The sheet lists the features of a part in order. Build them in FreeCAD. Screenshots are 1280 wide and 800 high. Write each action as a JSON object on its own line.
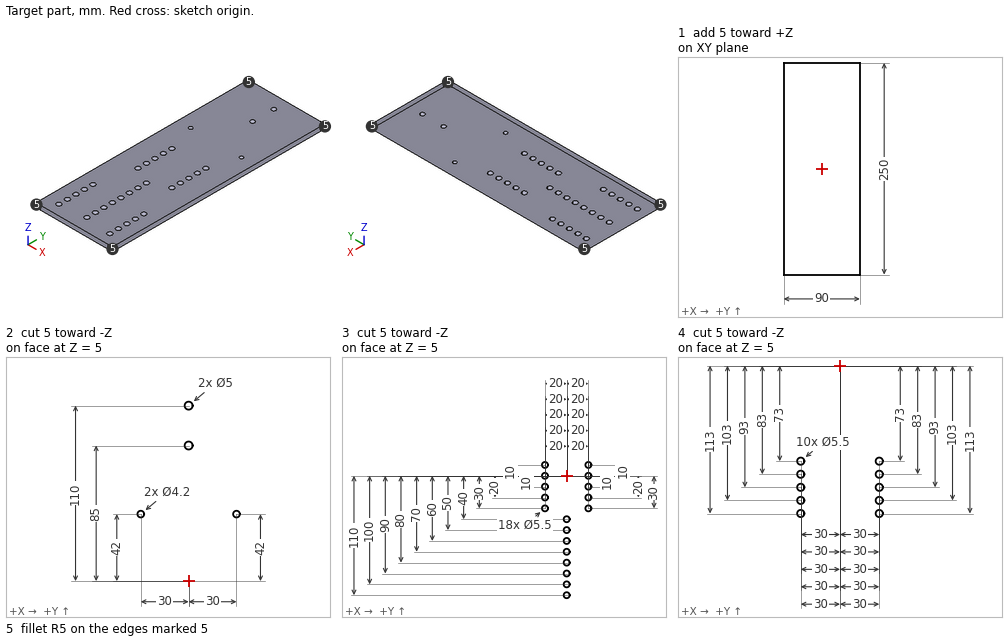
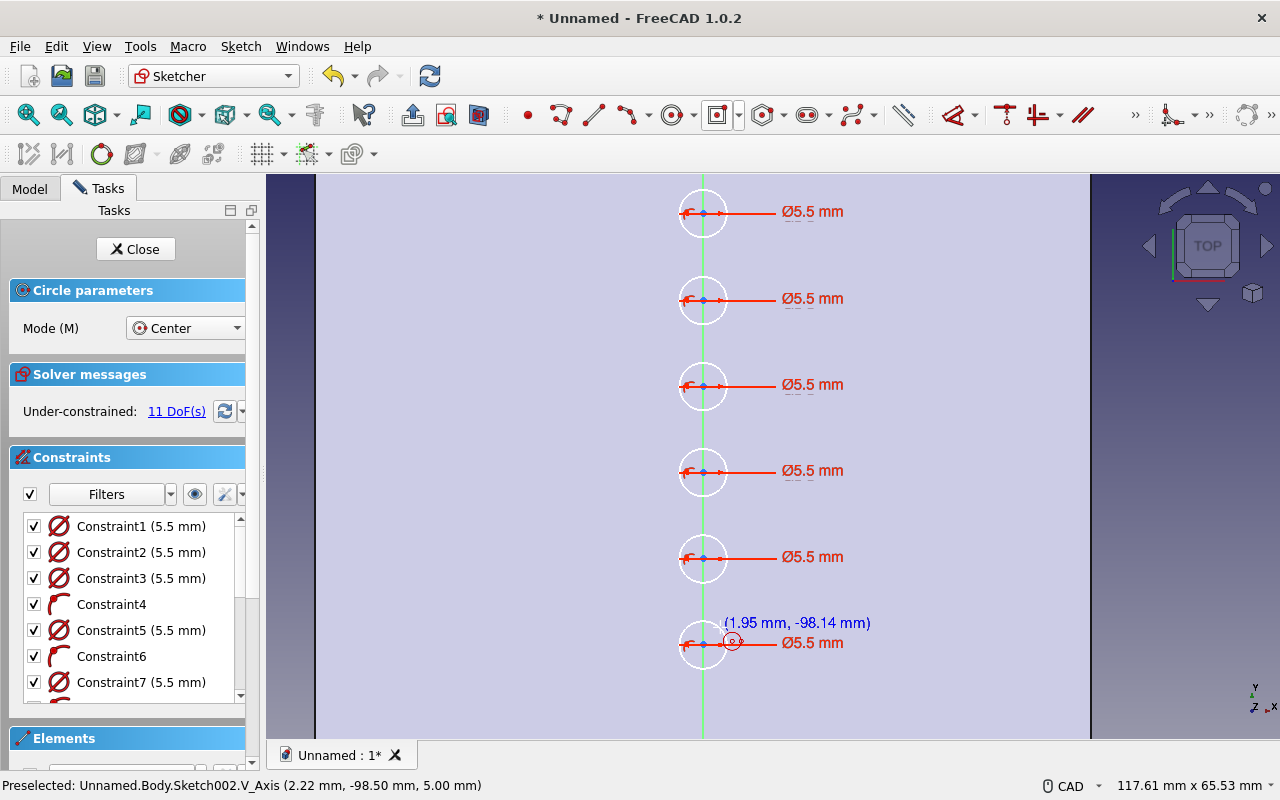
{"action": "scroll", "coordinate": [705, 561], "scroll_direction": "down", "scroll_amount": 6}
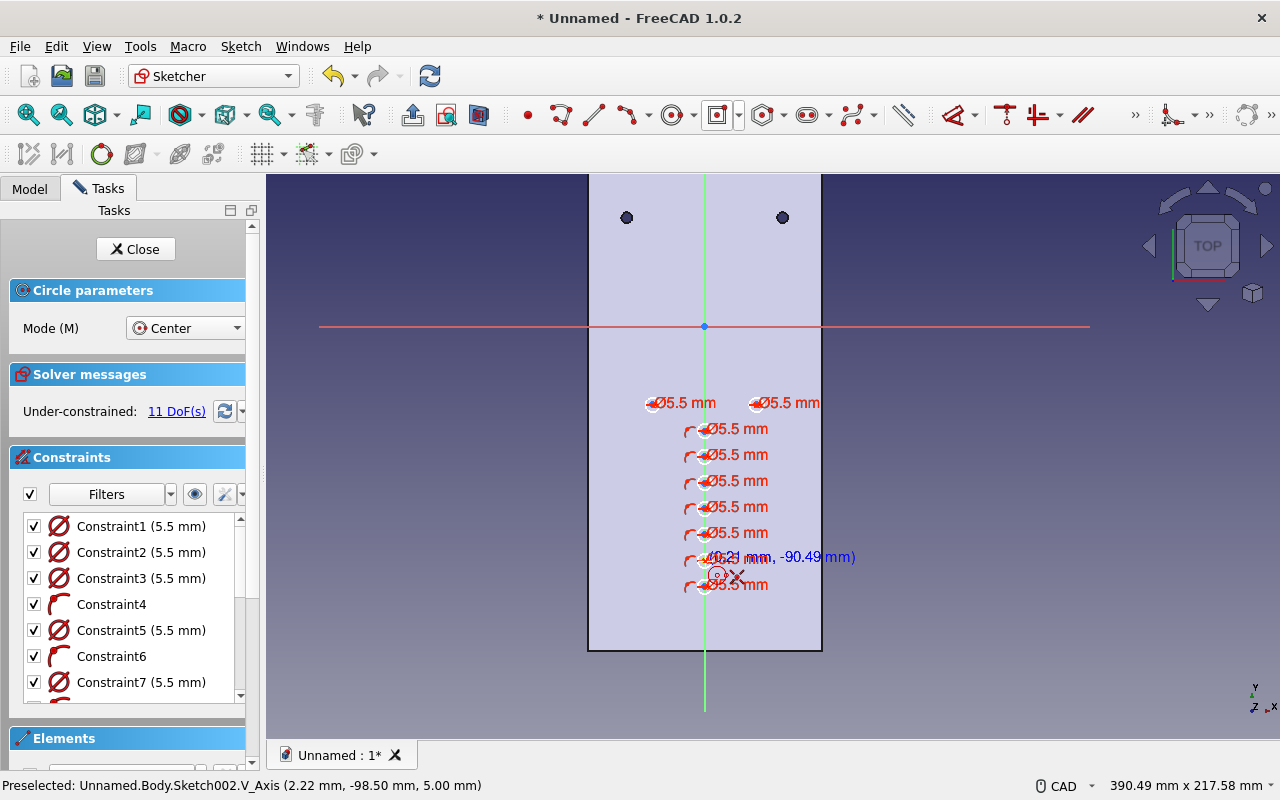
{"action": "scroll", "coordinate": [705, 612], "scroll_direction": "up", "scroll_amount": 6}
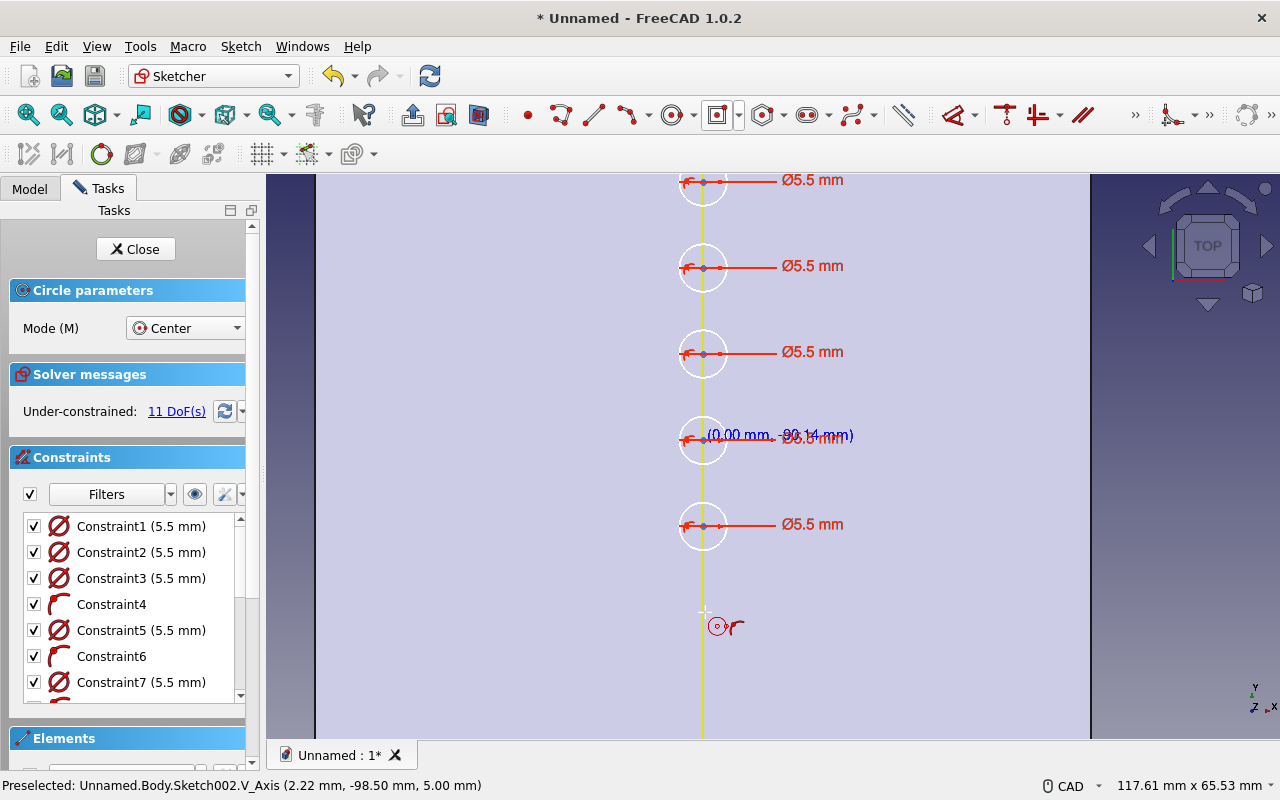
{"action": "left_click", "coordinate": [703, 612]}
{"action": "mouse_move", "coordinate": [720, 595]}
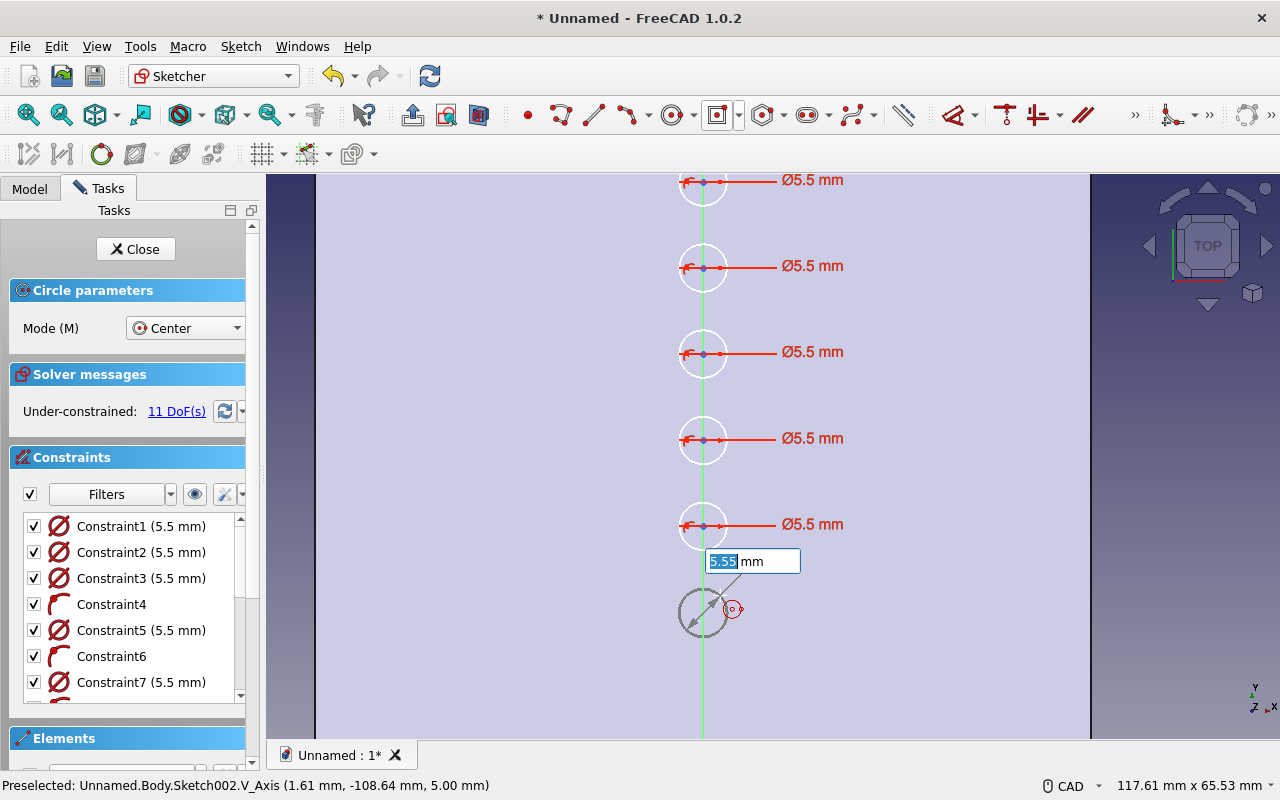
{"action": "type", "text": "5.5"}
{"action": "key", "text": "Return"}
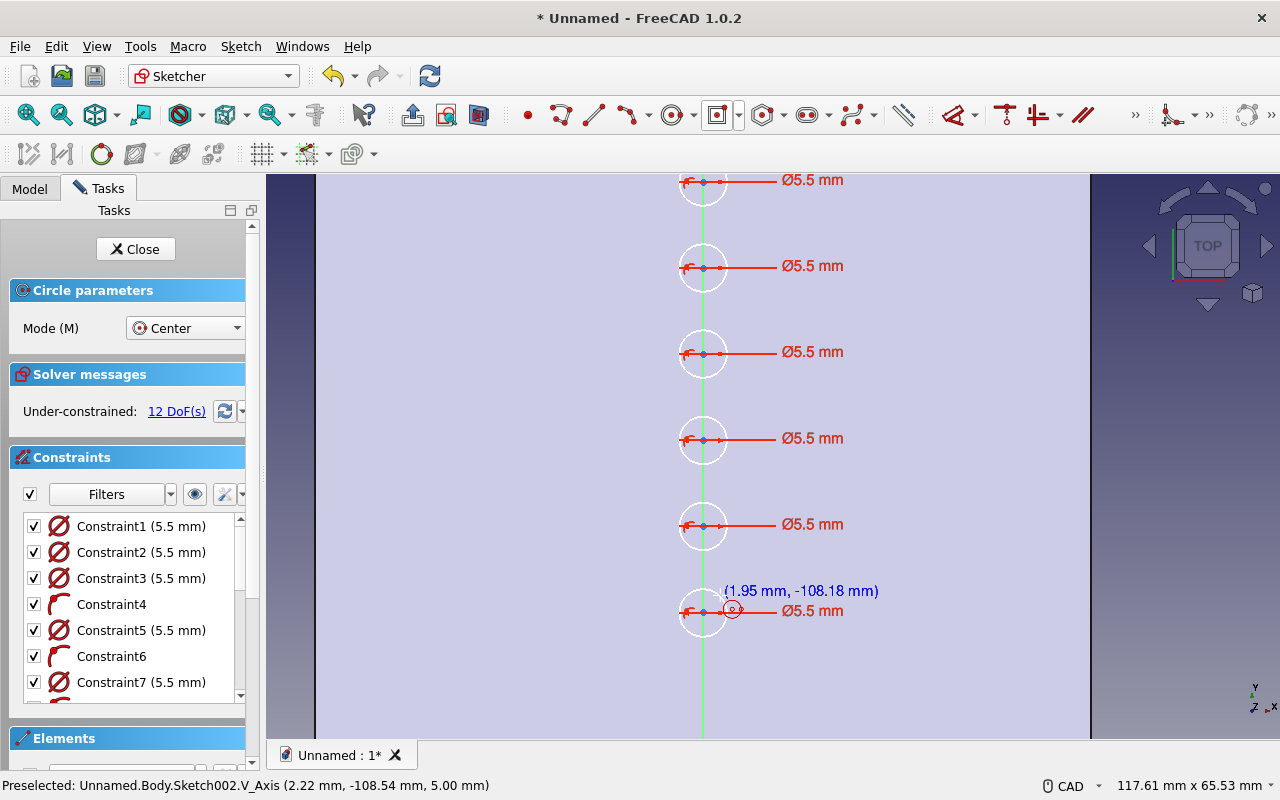
{"action": "scroll", "coordinate": [705, 613], "scroll_direction": "down", "scroll_amount": 6}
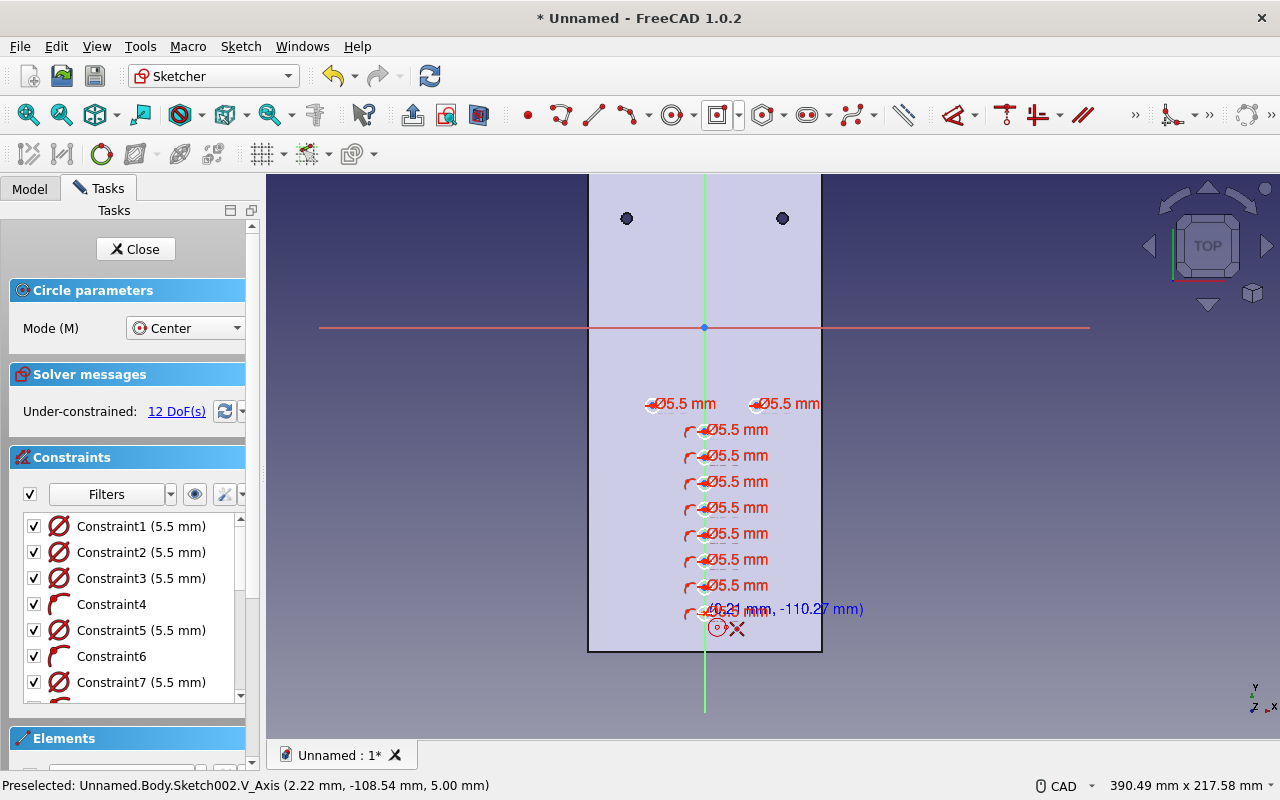
{"action": "scroll", "coordinate": [653, 379], "scroll_direction": "up", "scroll_amount": 6}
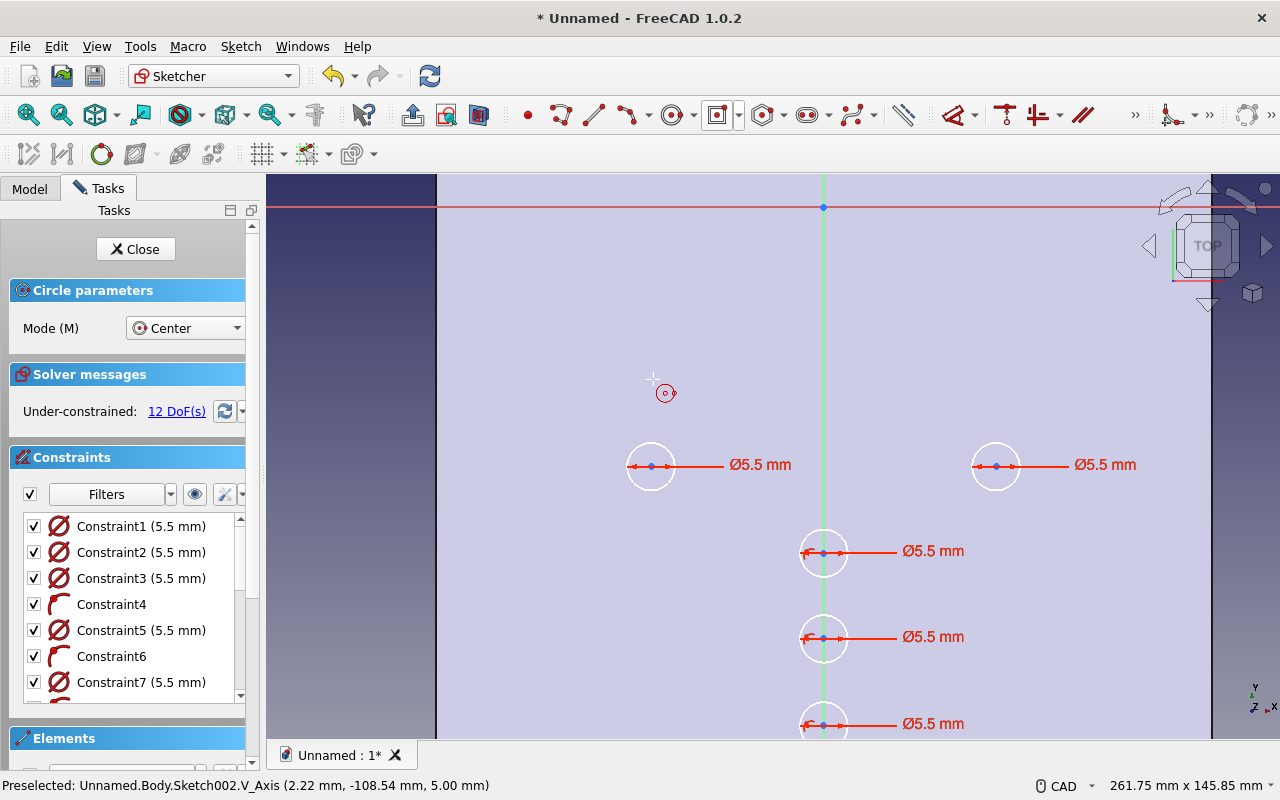
{"action": "left_click", "coordinate": [651, 380]}
{"action": "mouse_move", "coordinate": [668, 363]}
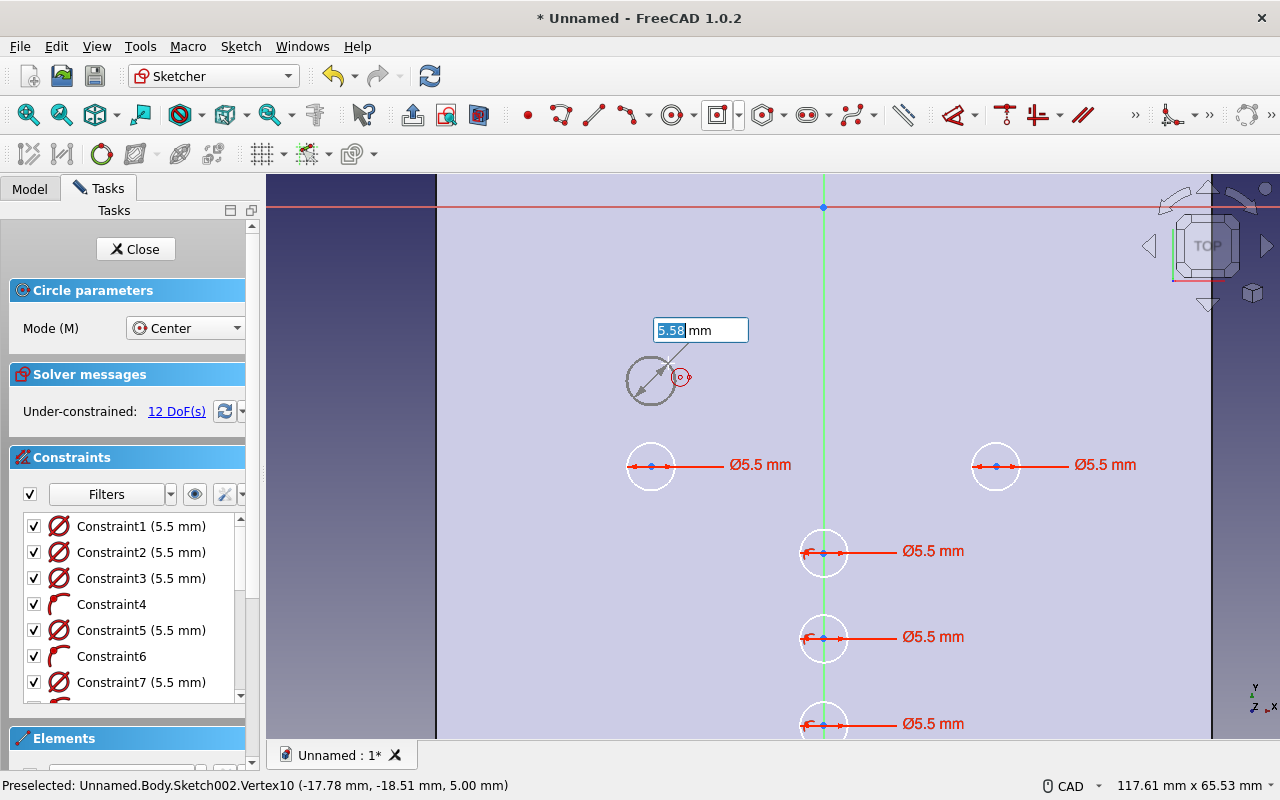
{"action": "type", "text": "5.5"}
{"action": "key", "text": "Return"}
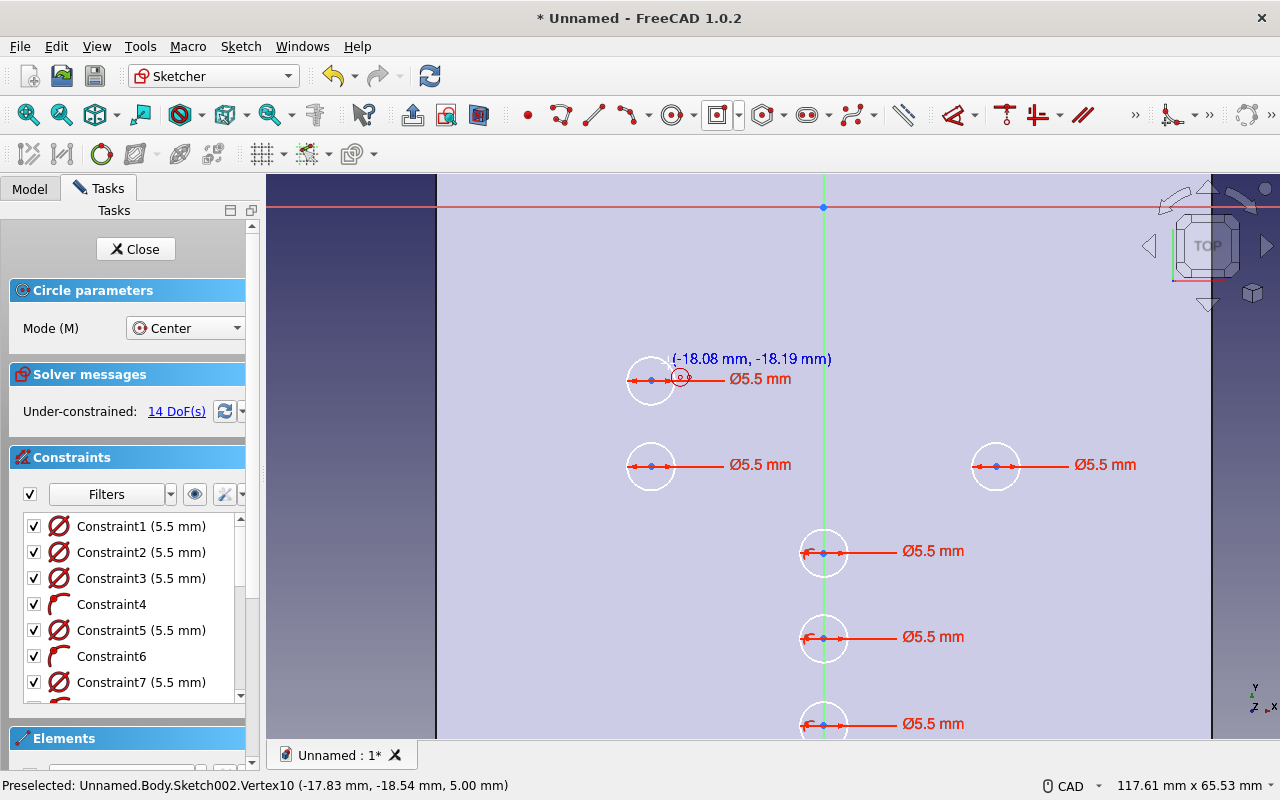
{"action": "left_click", "coordinate": [996, 380]}
{"action": "mouse_move", "coordinate": [1013, 363]}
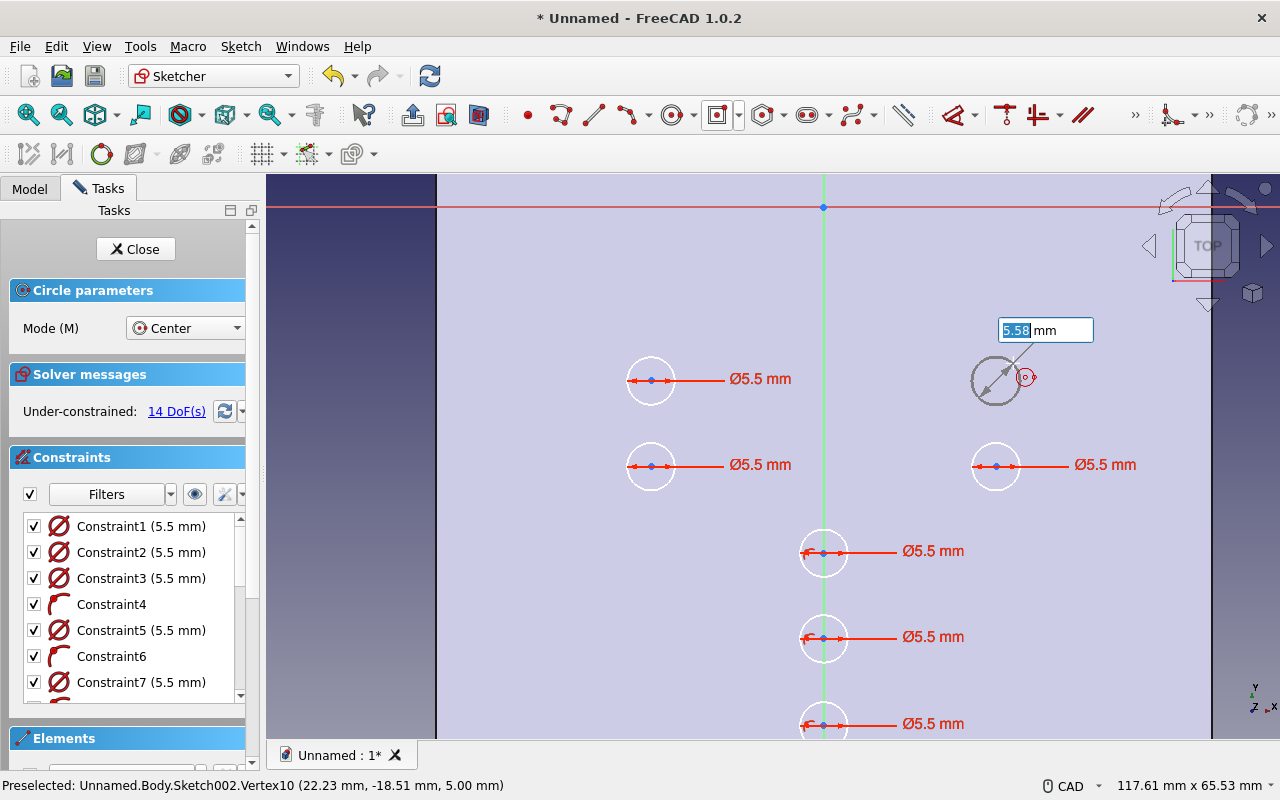
{"action": "type", "text": "5.5"}
{"action": "key", "text": "Return"}